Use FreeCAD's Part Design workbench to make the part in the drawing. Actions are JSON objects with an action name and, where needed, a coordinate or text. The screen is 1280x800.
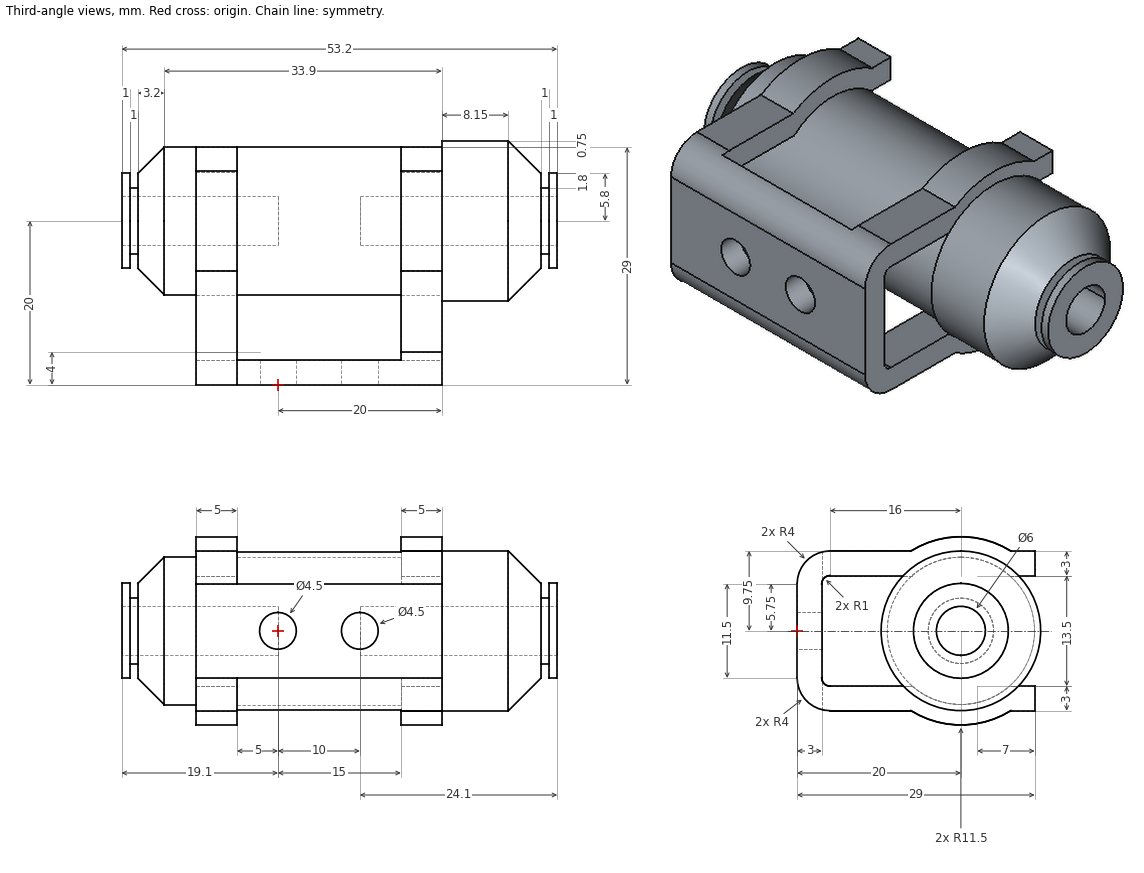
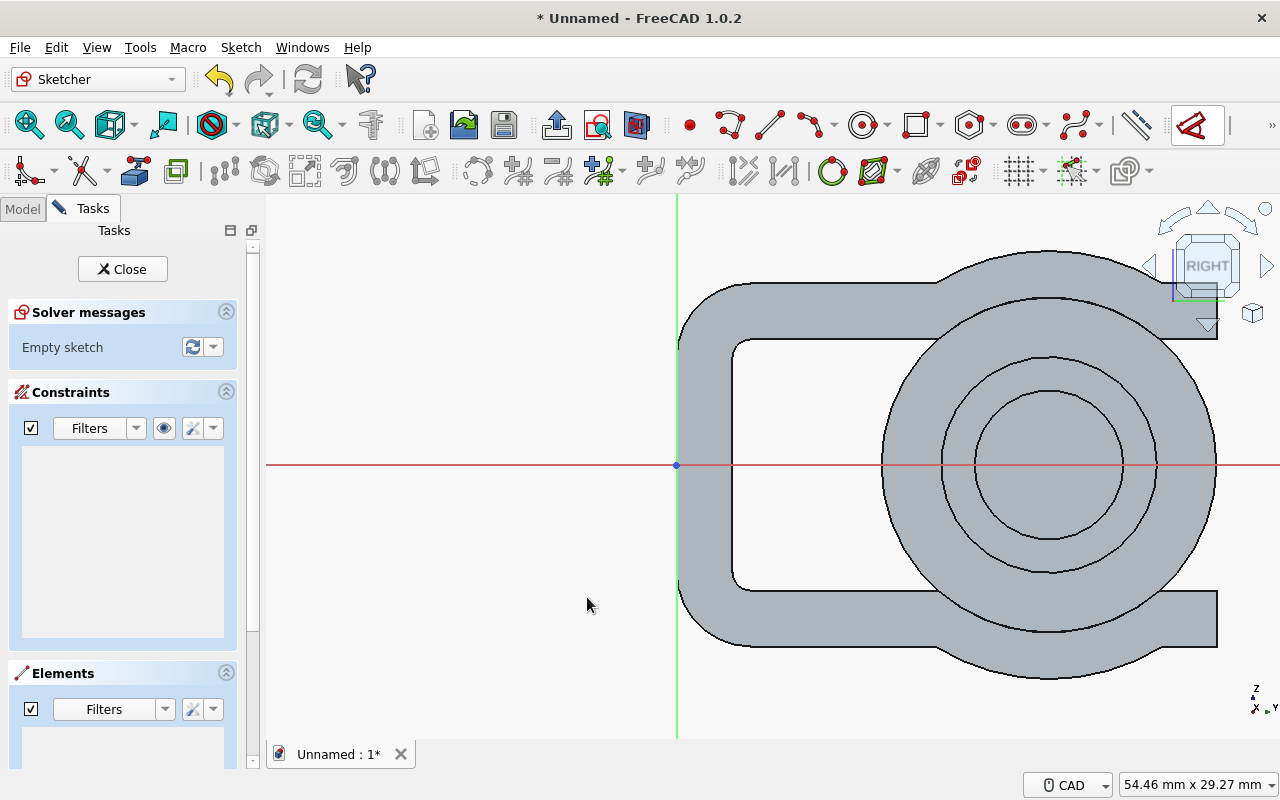
{"action": "left_click", "coordinate": [770, 126]}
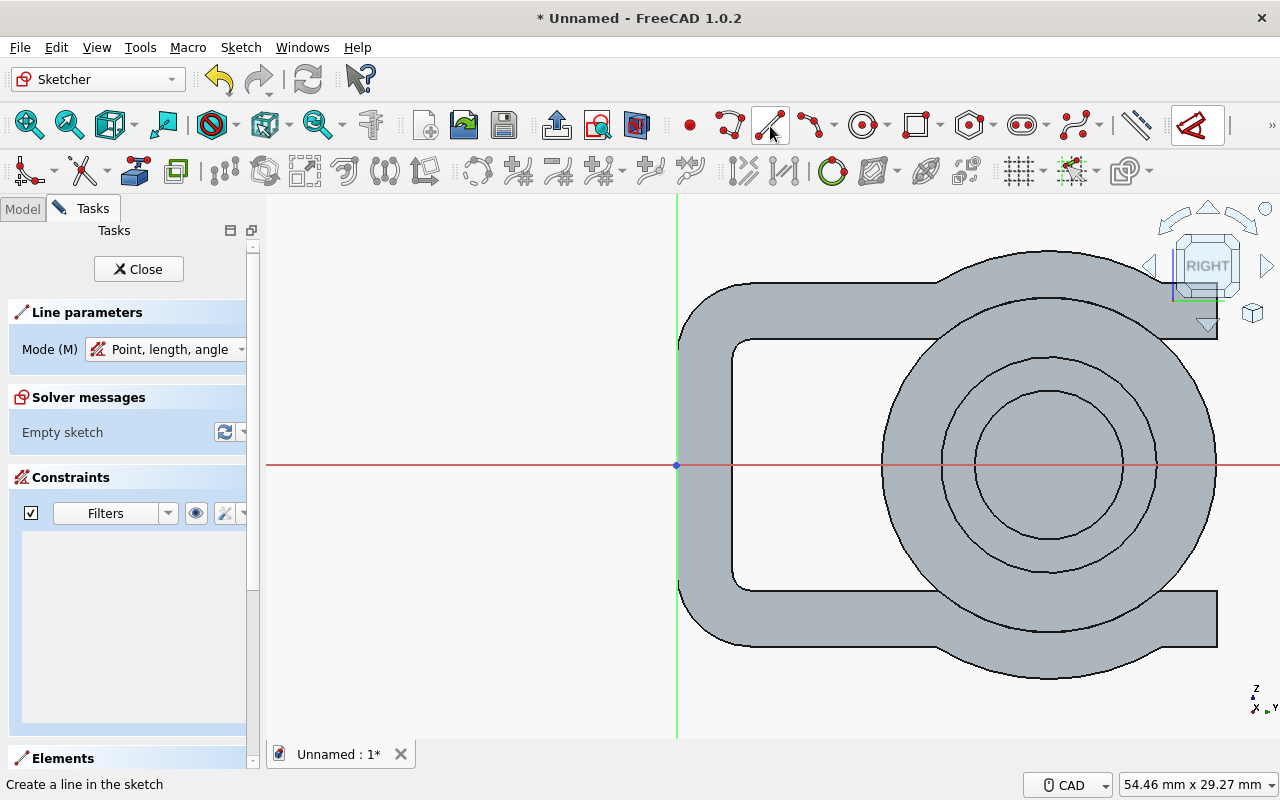
{"action": "left_click", "coordinate": [677, 358]}
{"action": "left_click", "coordinate": [686, 572]}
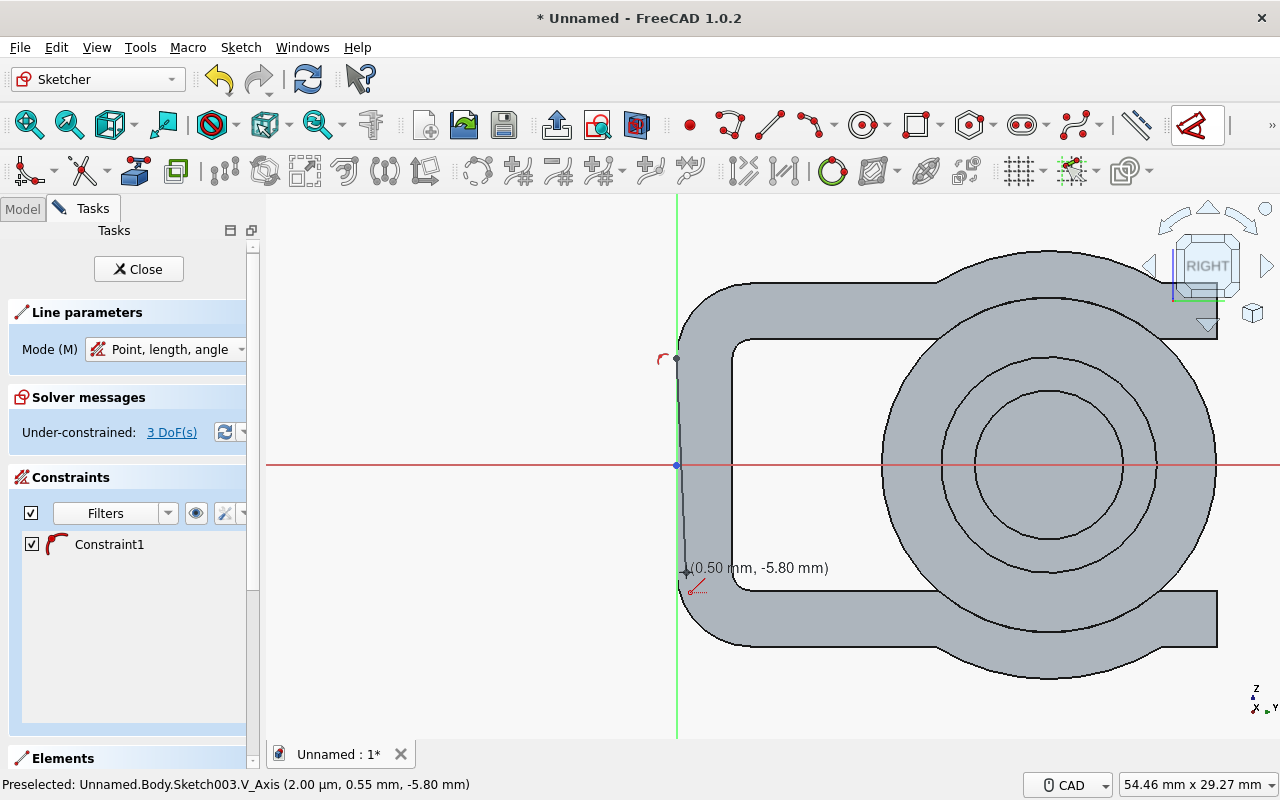
{"action": "left_click", "coordinate": [732, 644]}
{"action": "left_click", "coordinate": [732, 286]}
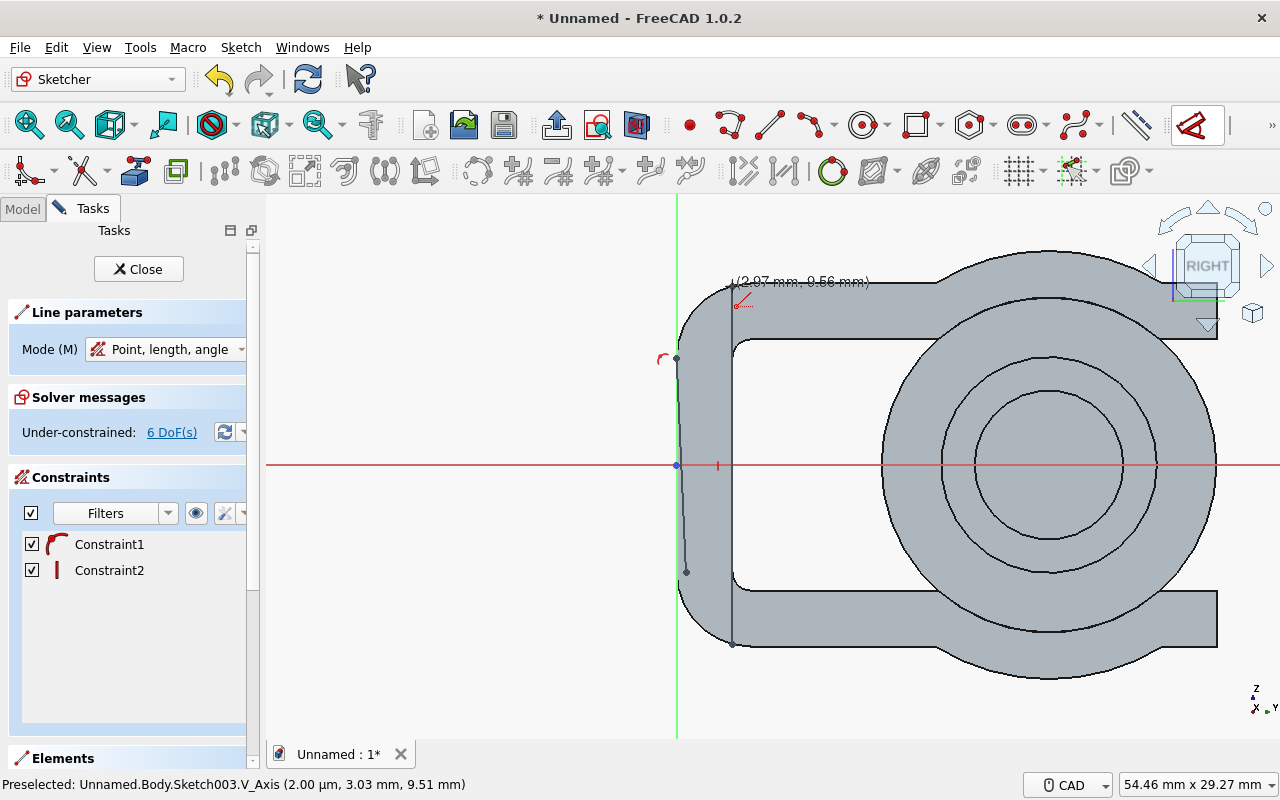
{"action": "left_click", "coordinate": [810, 126]}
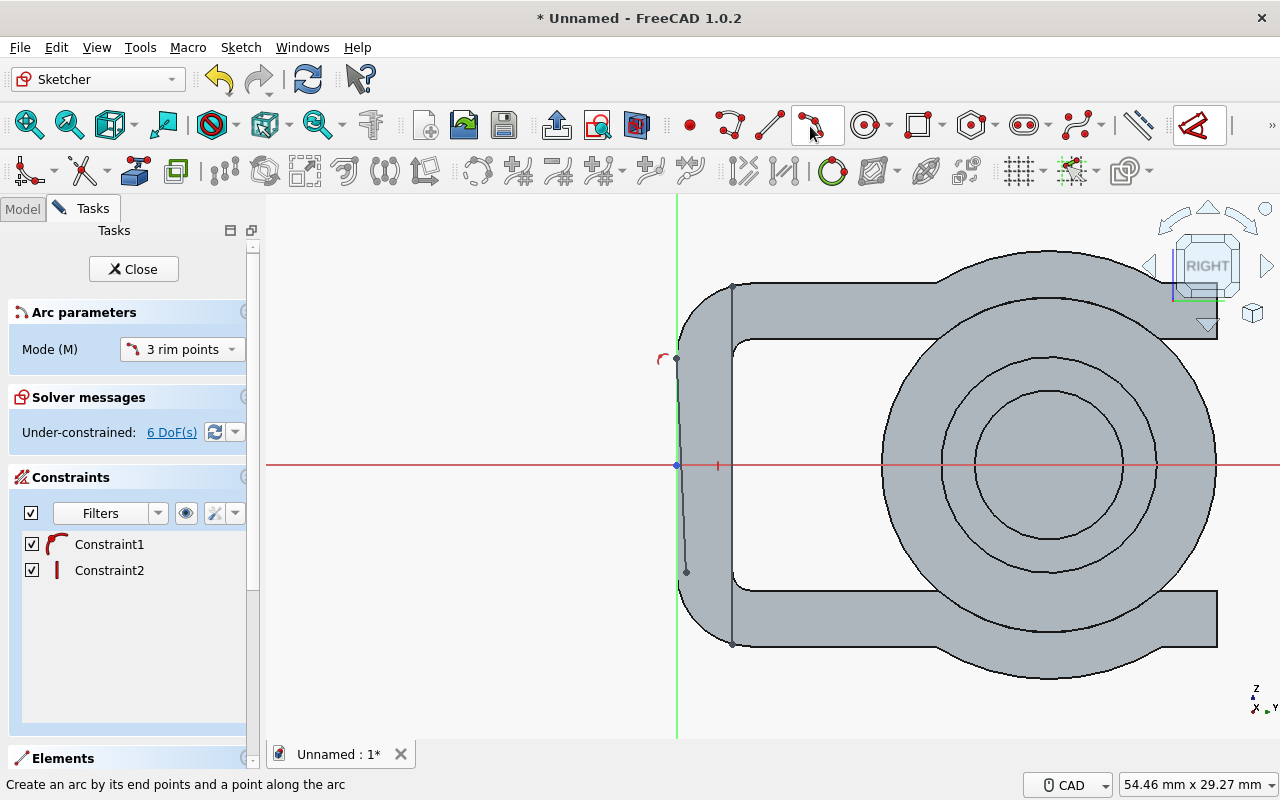
{"action": "left_click", "coordinate": [686, 573]}
{"action": "left_click", "coordinate": [732, 645]}
{"action": "left_click", "coordinate": [692, 618]}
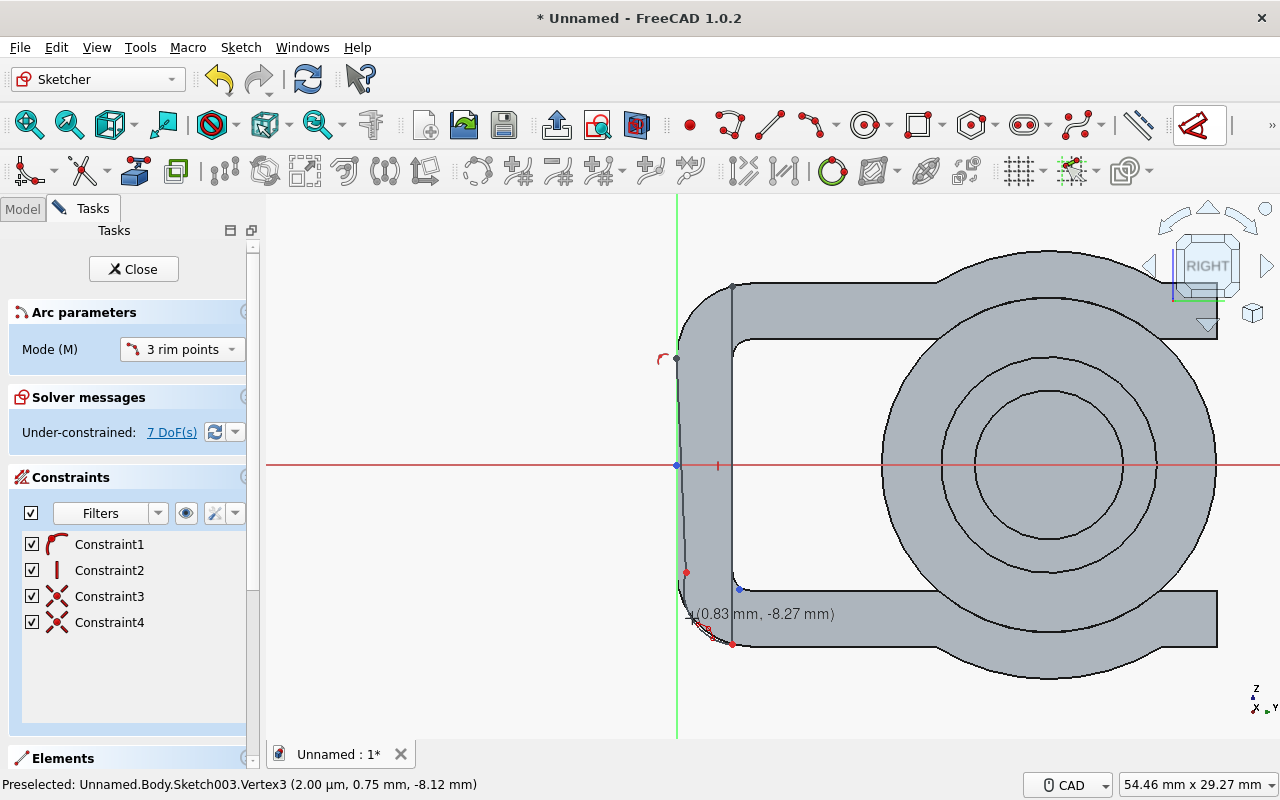
{"action": "left_click", "coordinate": [732, 287]}
{"action": "left_click", "coordinate": [677, 359]}
{"action": "left_click", "coordinate": [692, 312]}
{"action": "key", "text": "Escape"}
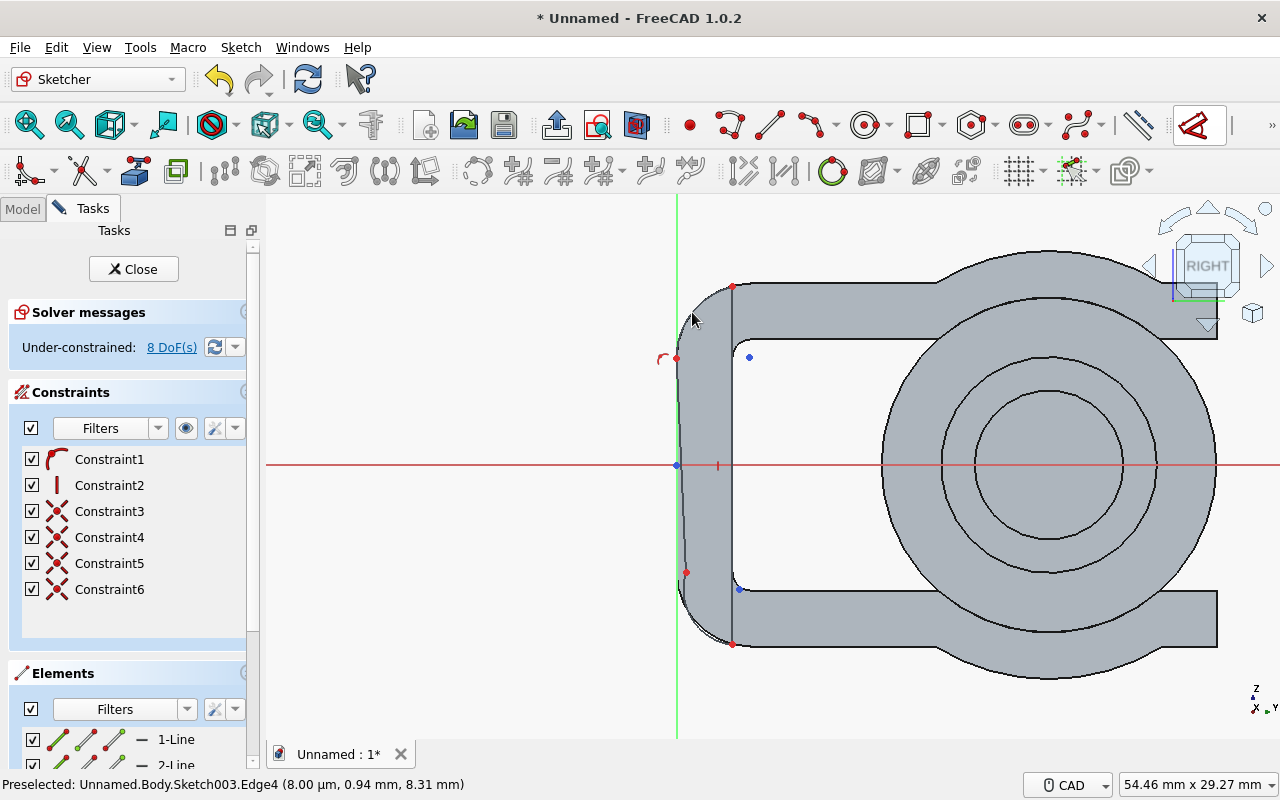
{"action": "left_click", "coordinate": [679, 423]}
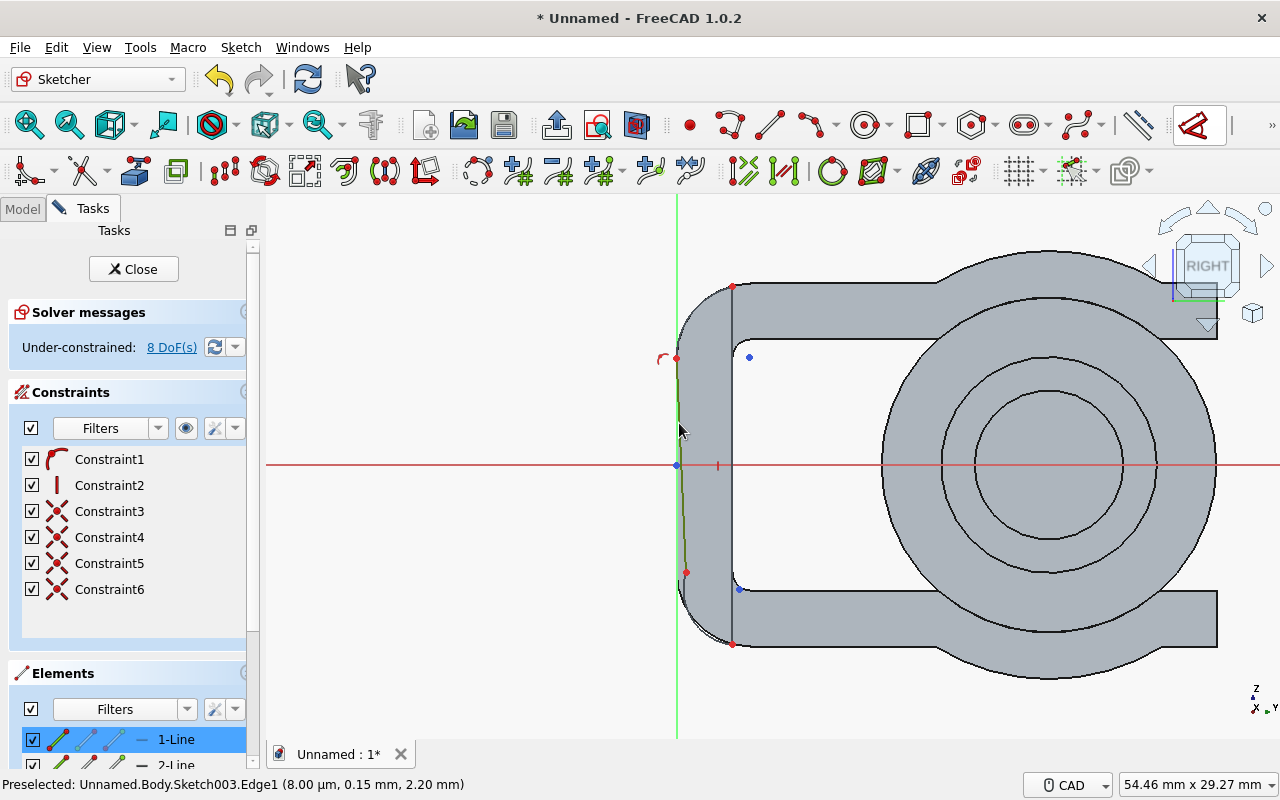
{"action": "left_click", "coordinate": [705, 634]}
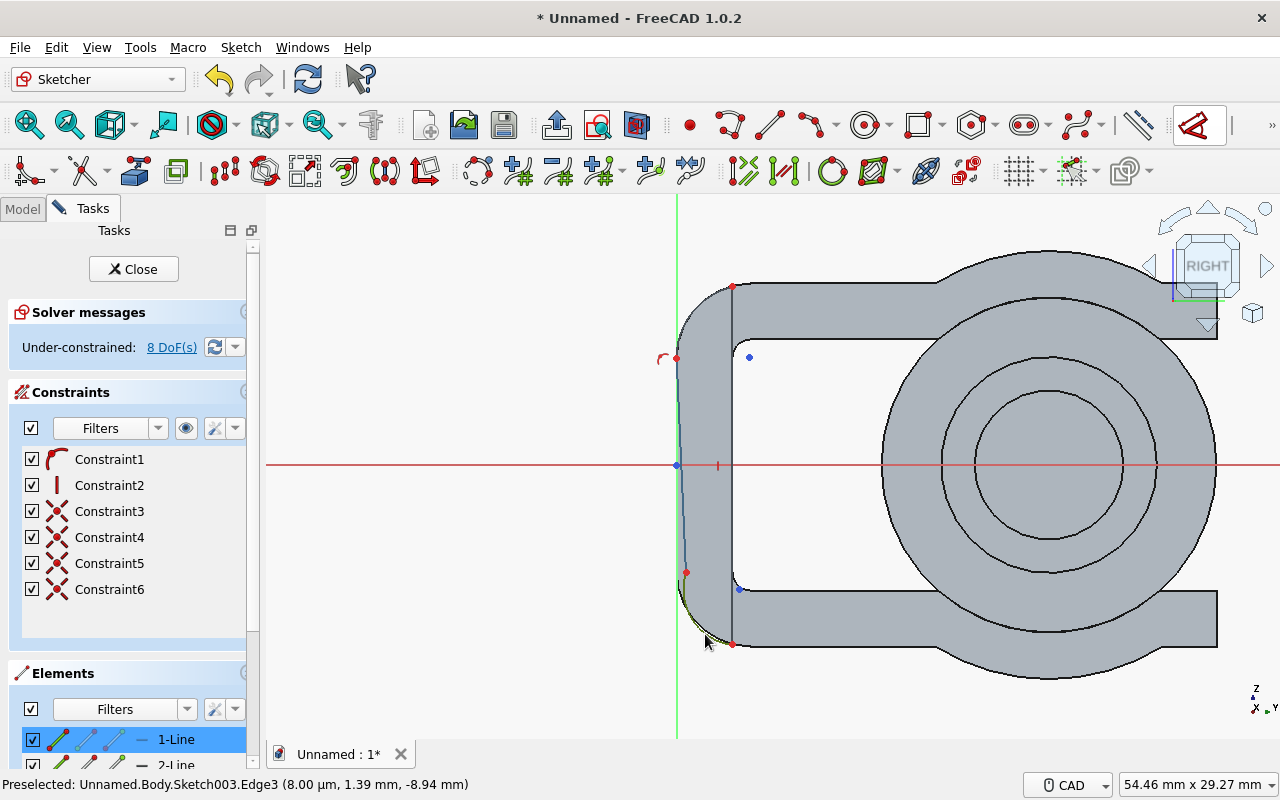
{"action": "key", "text": "t"}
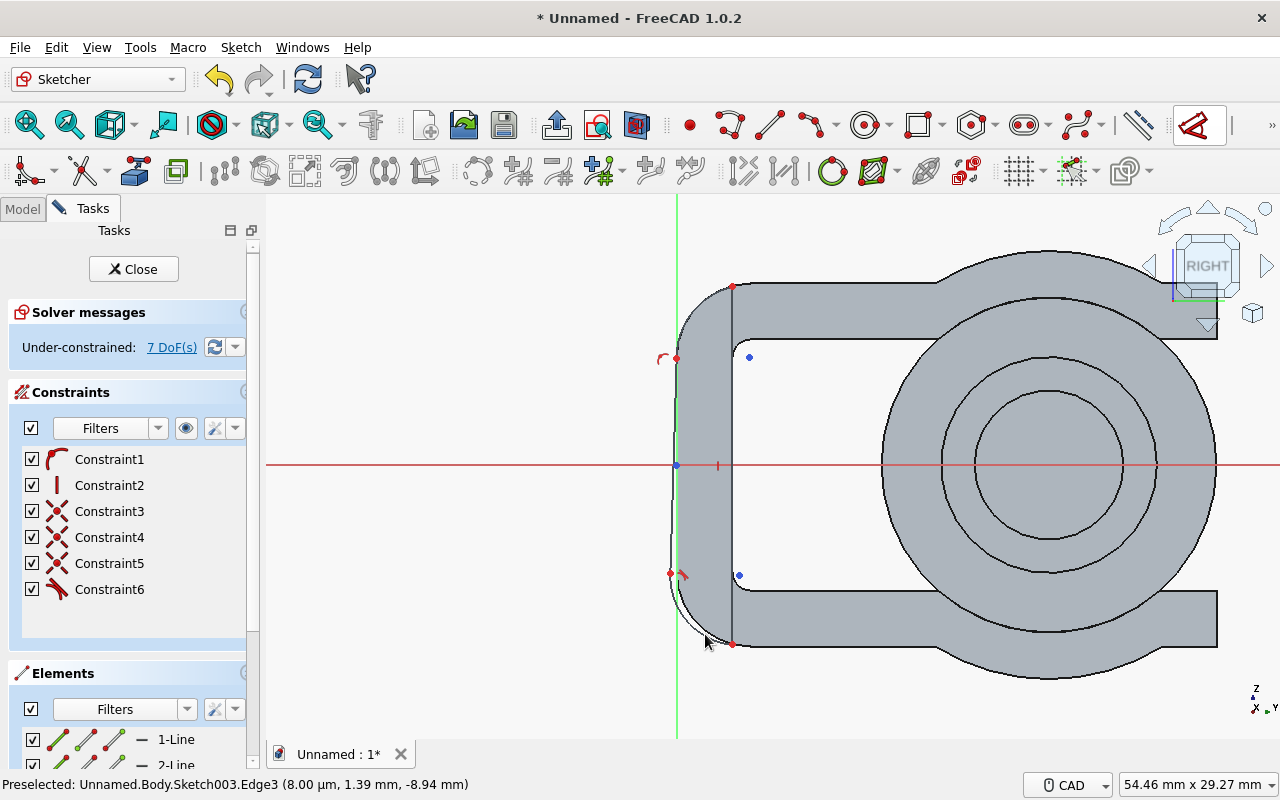
{"action": "left_click", "coordinate": [675, 423]}